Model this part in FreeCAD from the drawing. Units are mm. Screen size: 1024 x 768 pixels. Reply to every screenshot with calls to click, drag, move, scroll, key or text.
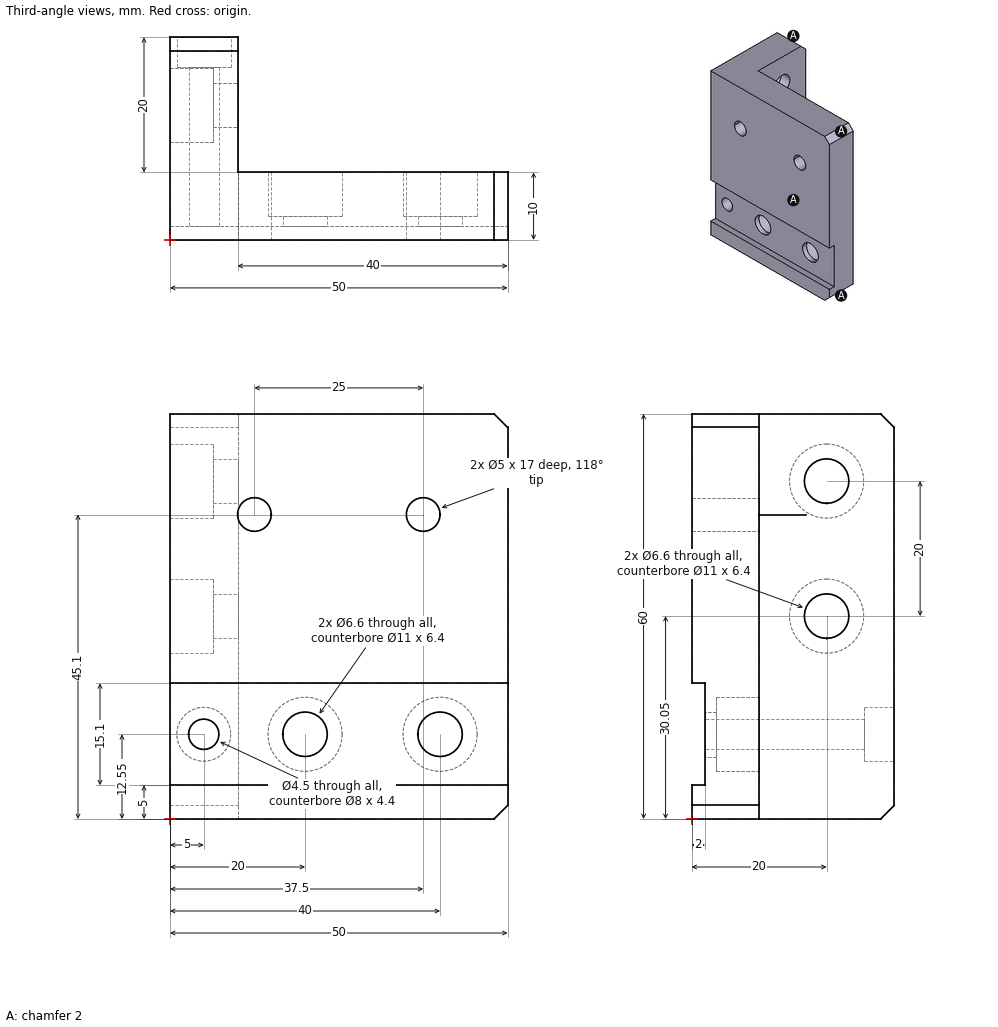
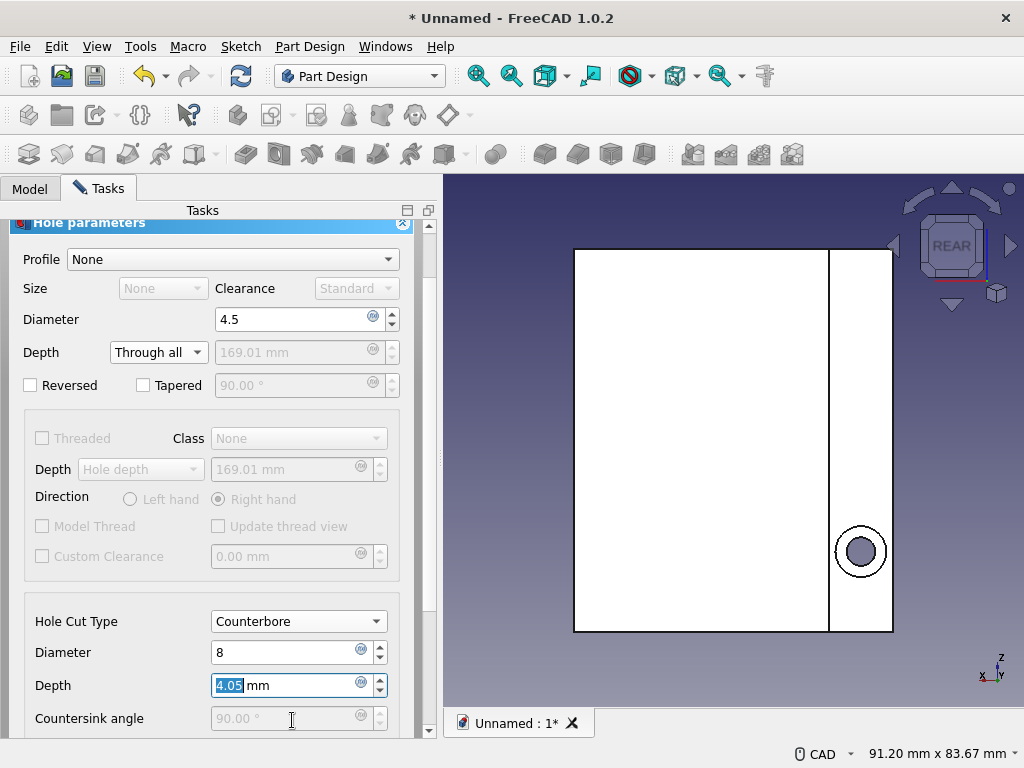
text(4.4)
key(Tab)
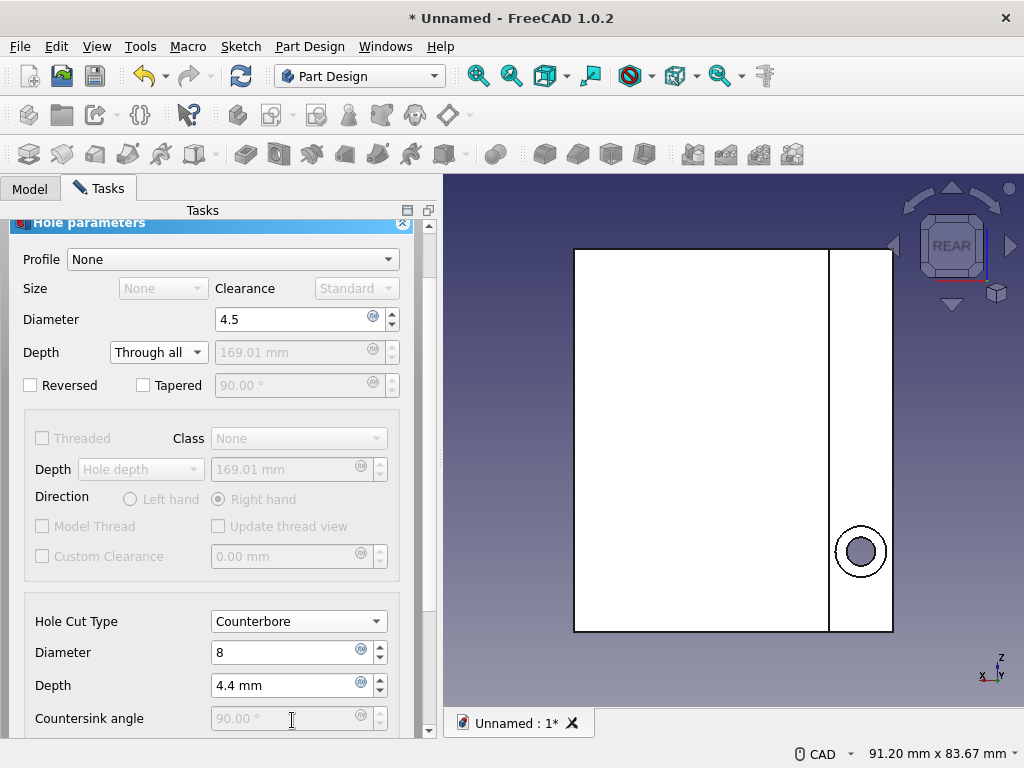
scroll(429, 479, up, 2)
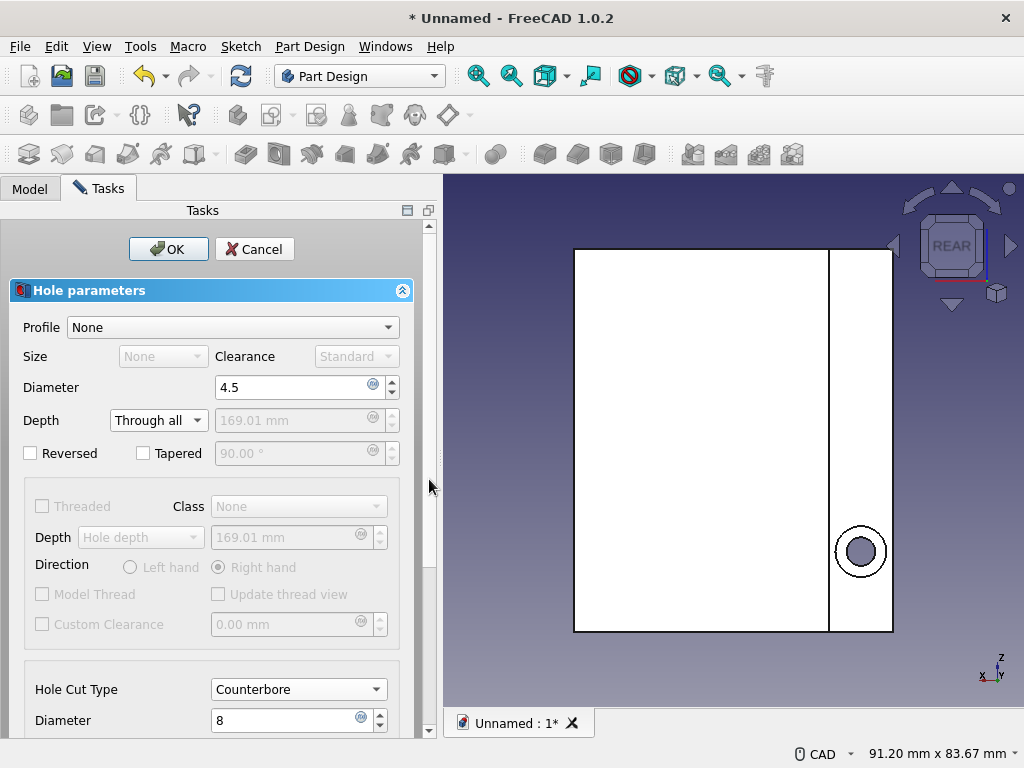
click(169, 249)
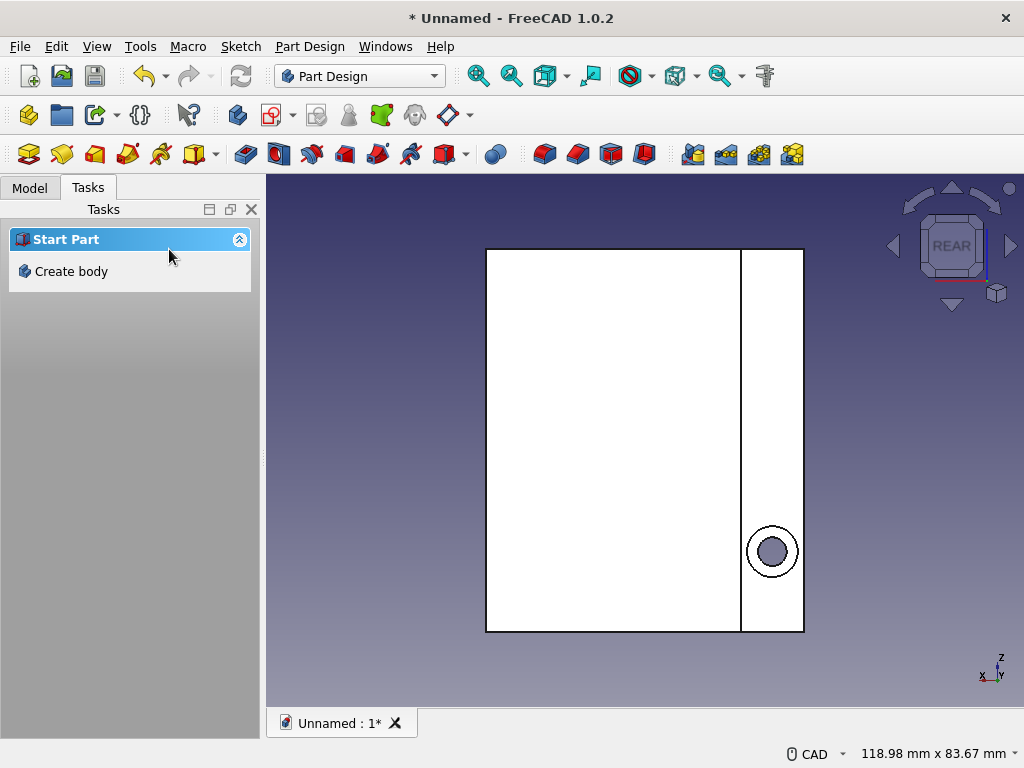
click(613, 385)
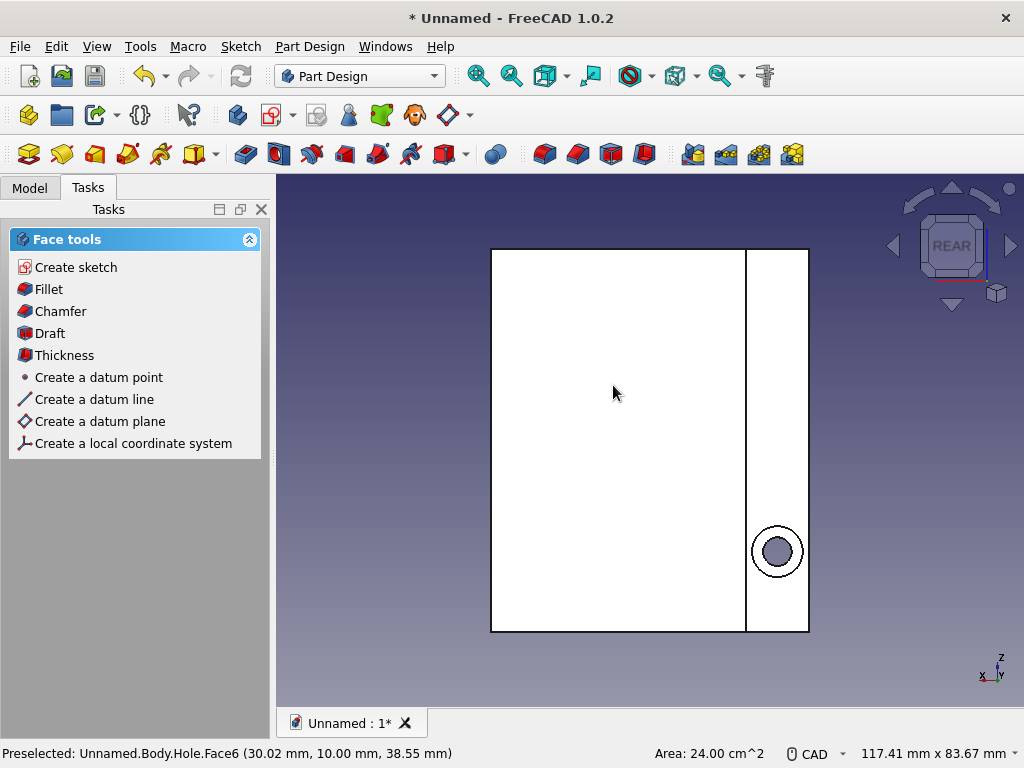
click(270, 116)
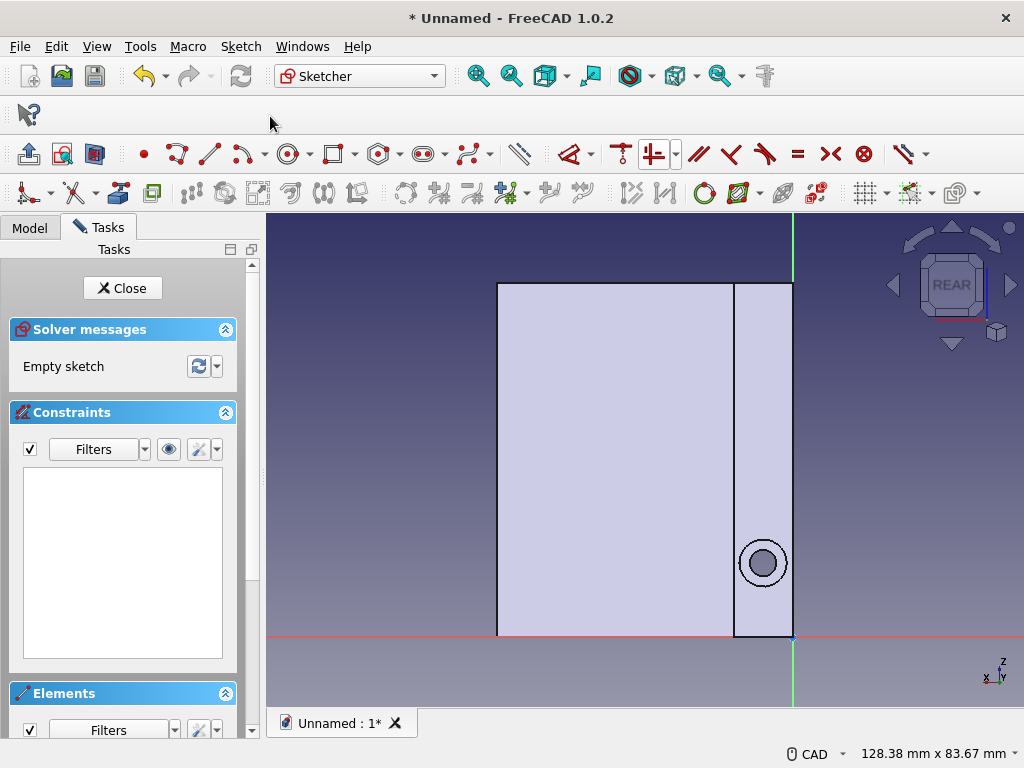
scroll(844, 679, up, 2)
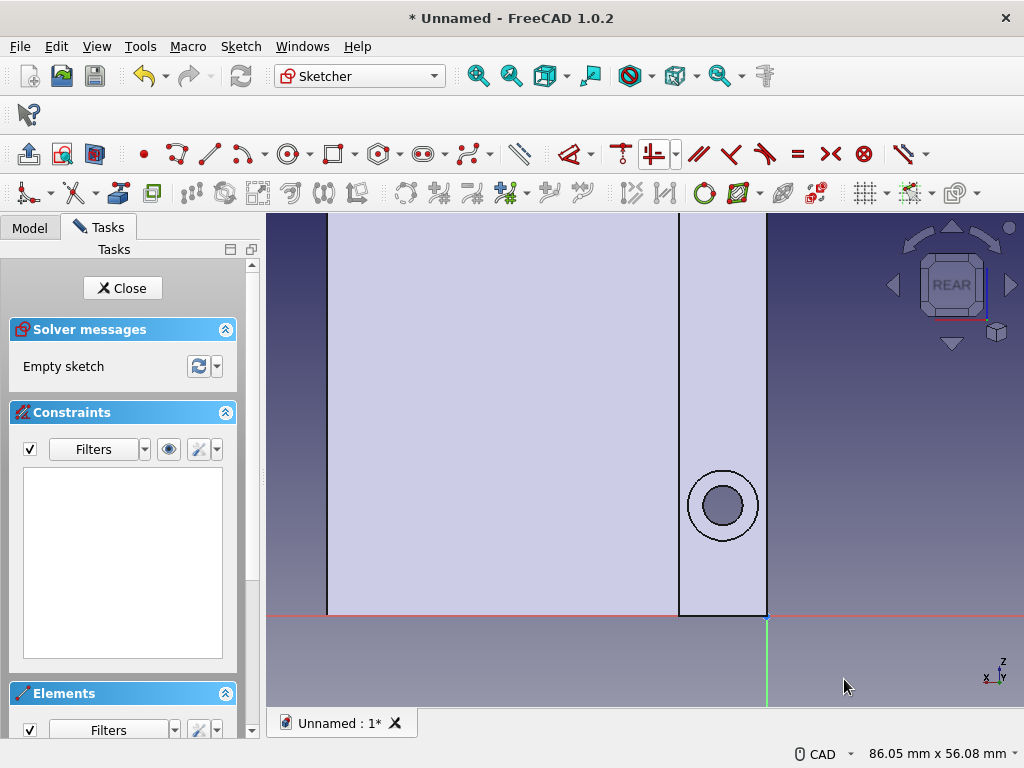
click(288, 154)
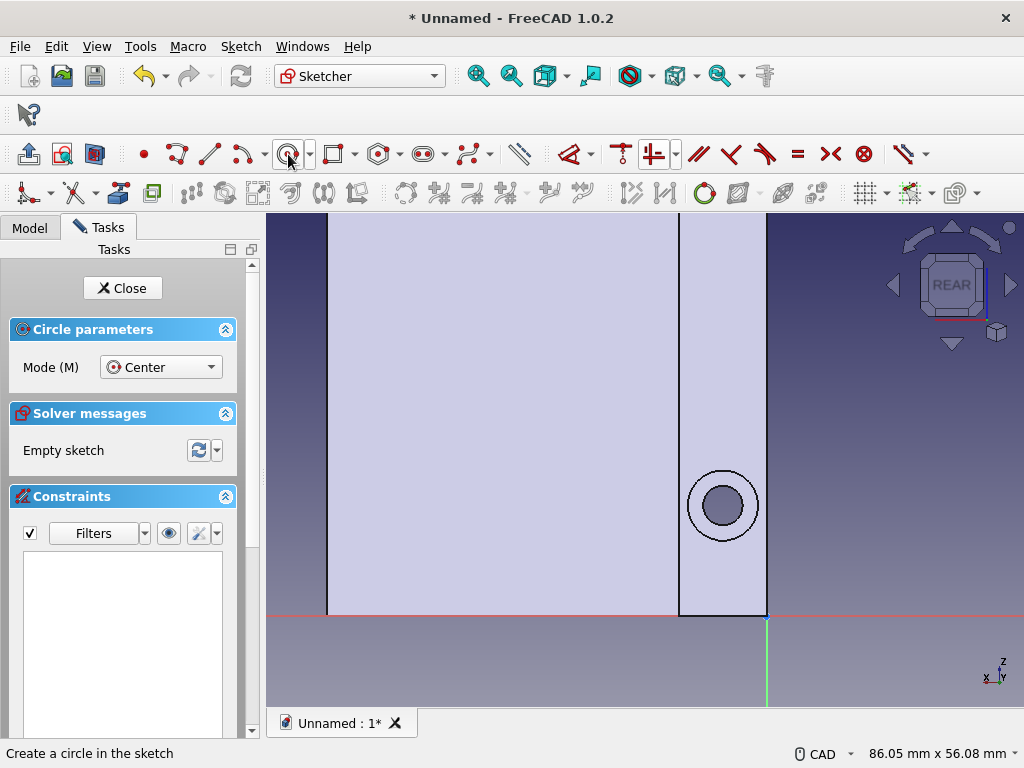
click(591, 506)
click(611, 485)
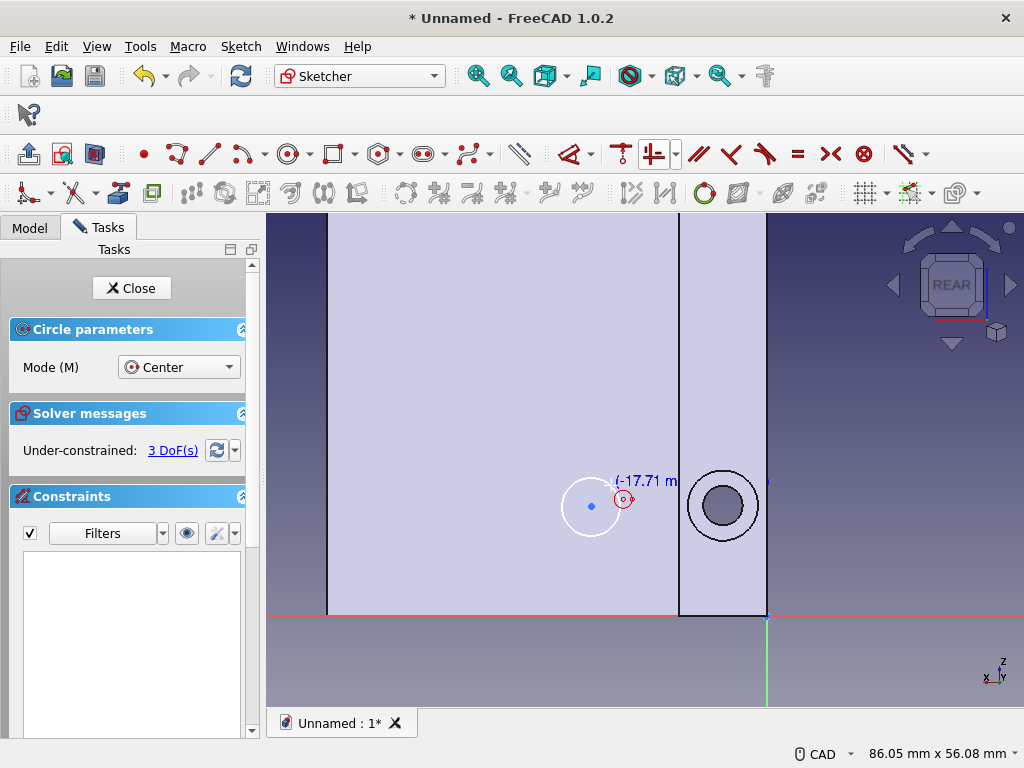
click(415, 506)
click(435, 485)
key(Escape)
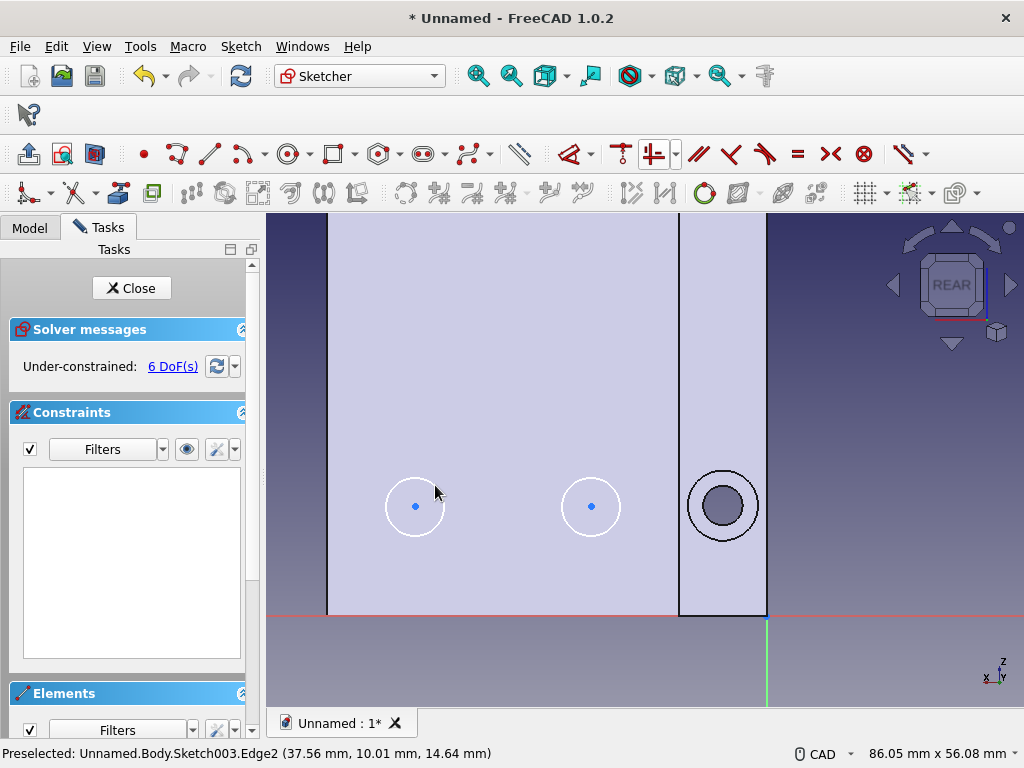
click(611, 486)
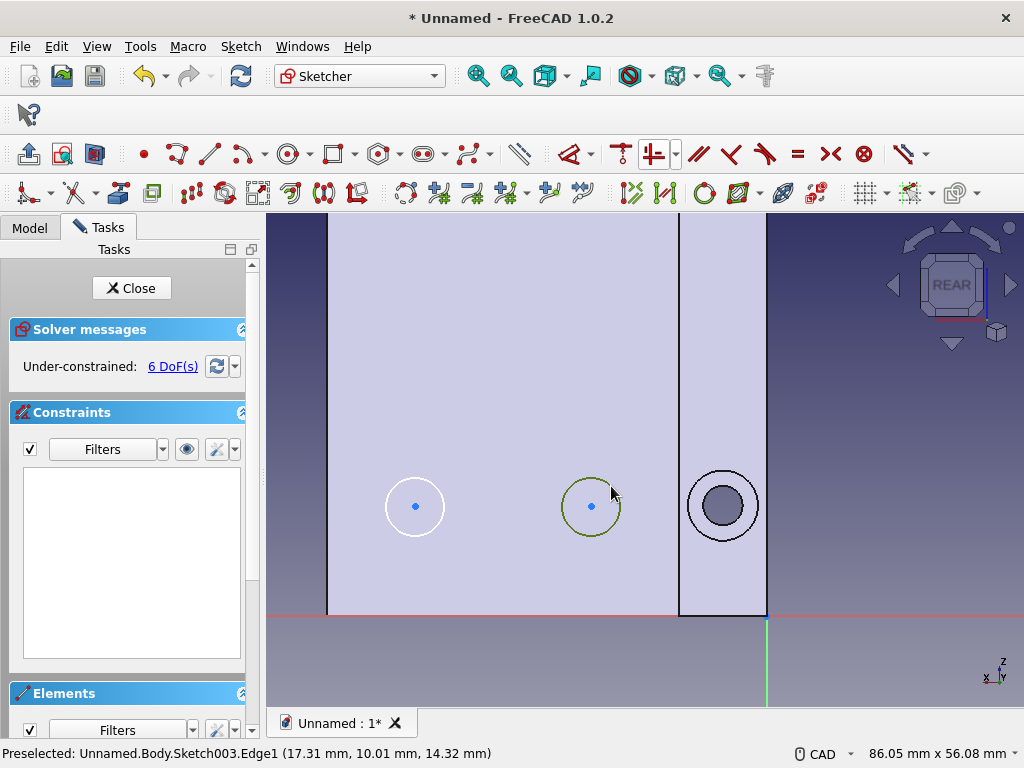
click(435, 486)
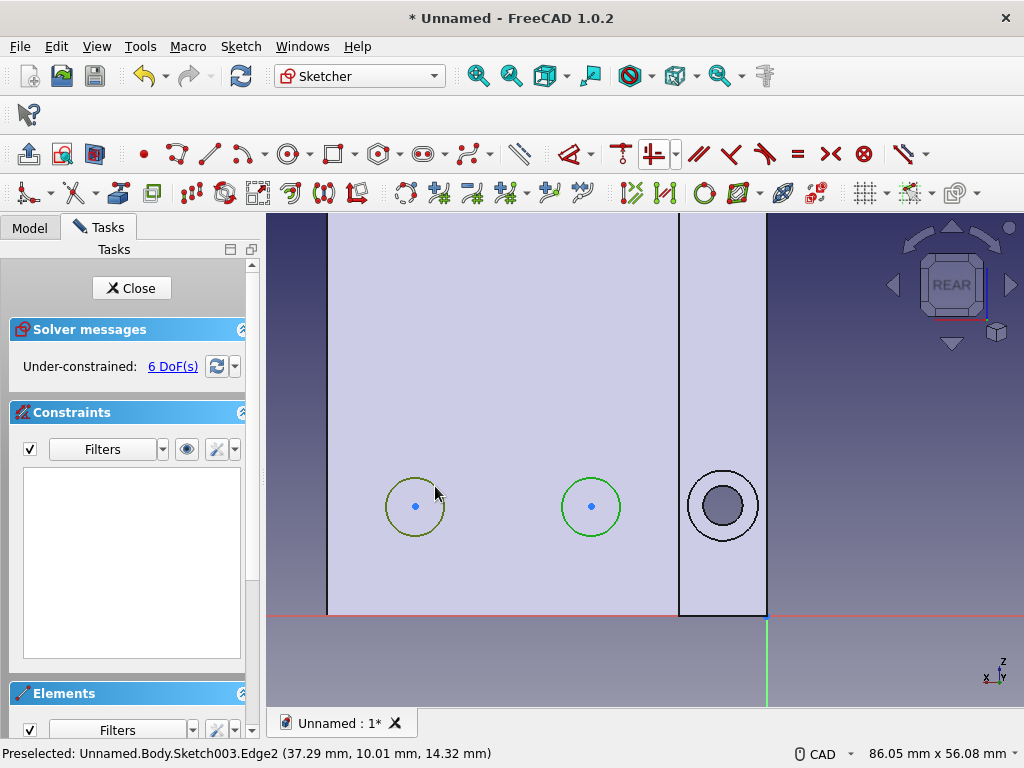
click(798, 154)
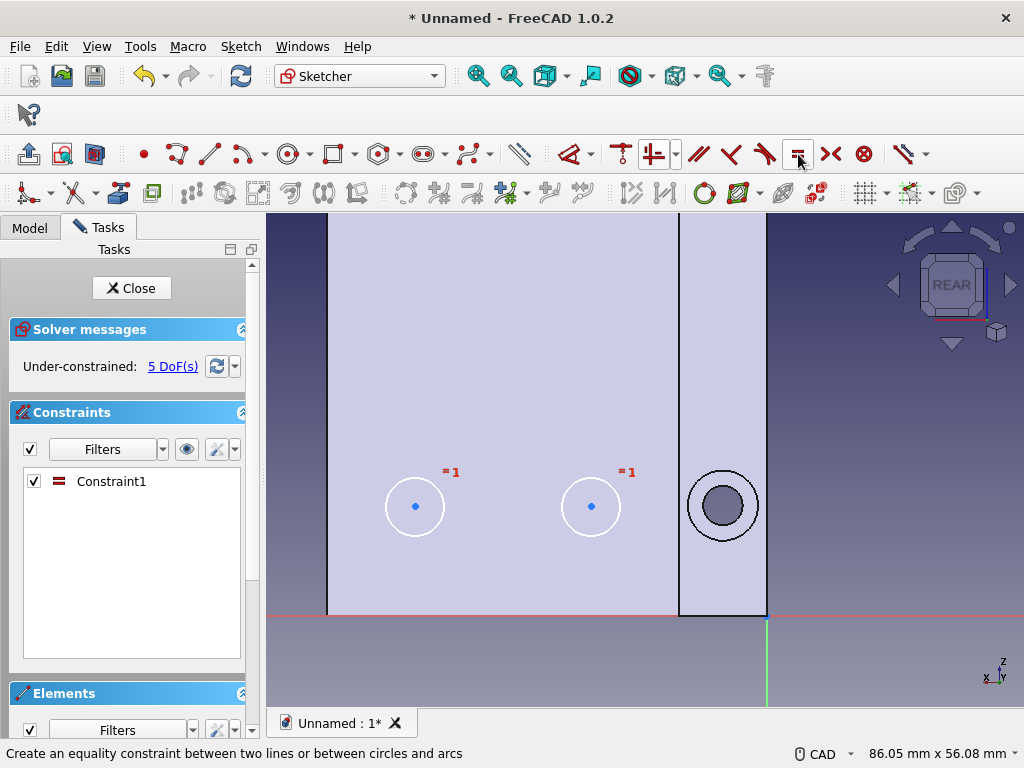
click(568, 154)